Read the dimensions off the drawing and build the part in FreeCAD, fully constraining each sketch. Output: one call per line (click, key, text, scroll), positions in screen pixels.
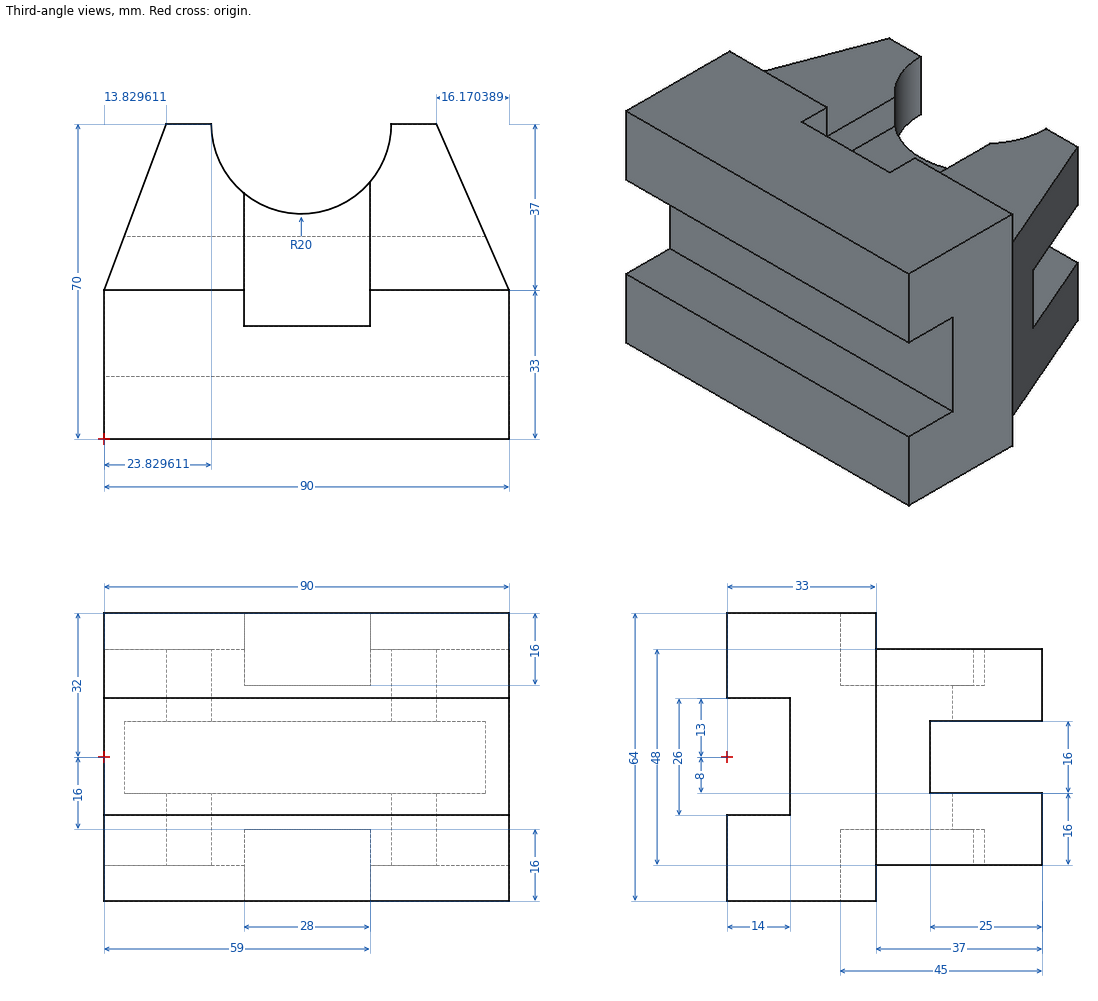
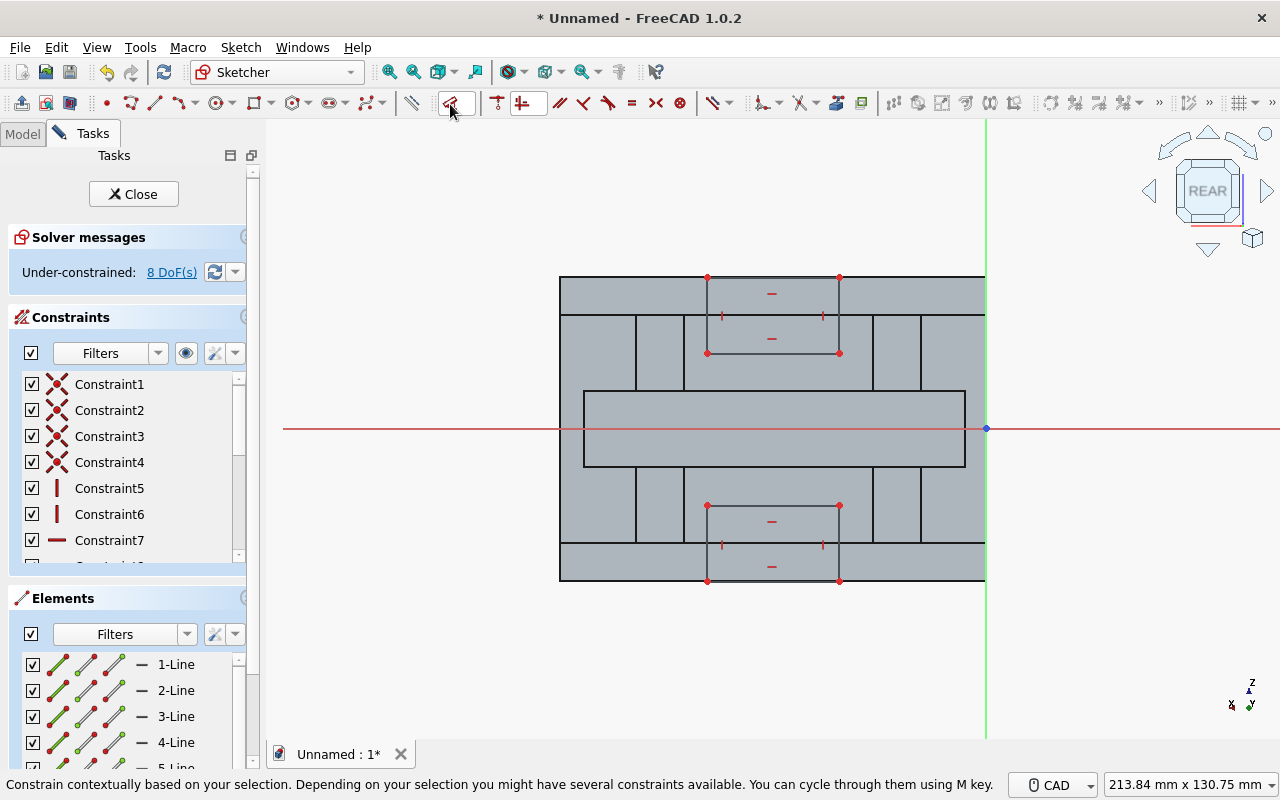
click(707, 529)
click(673, 544)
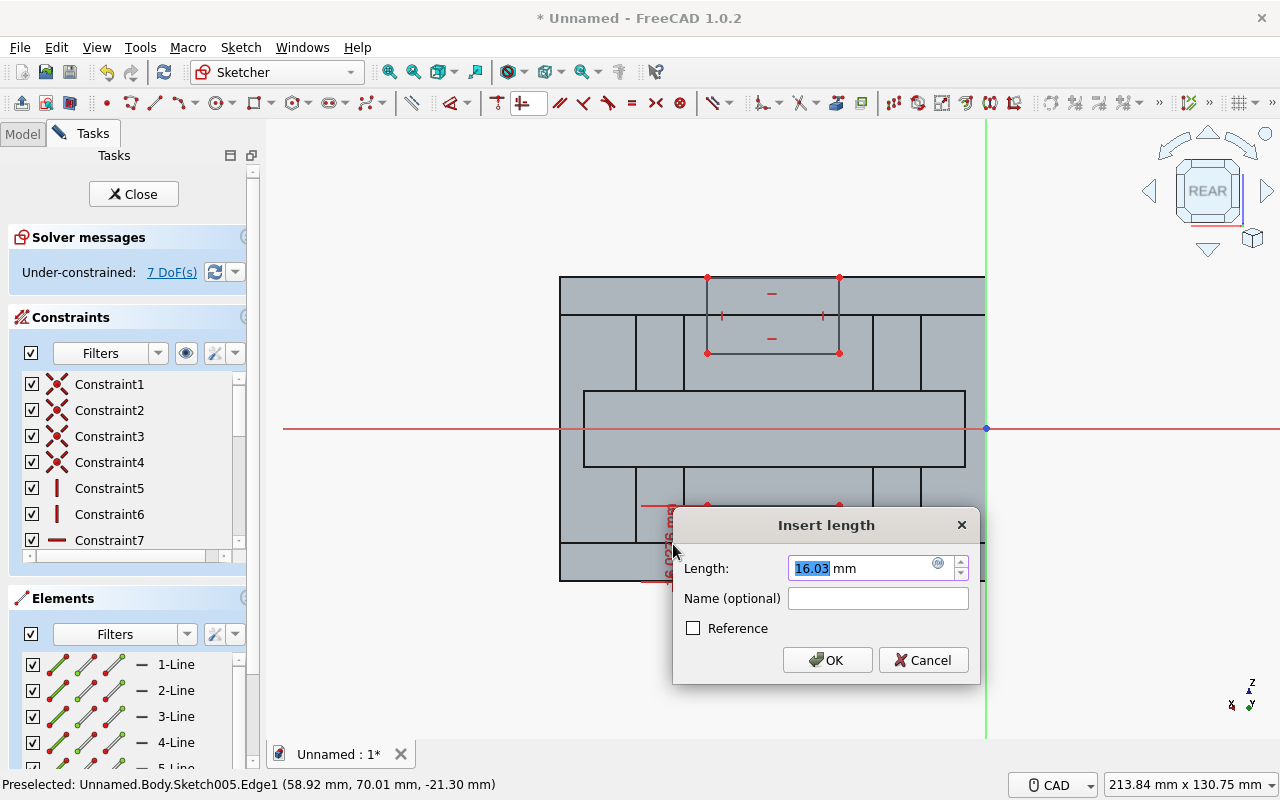
text(16)
key(Return)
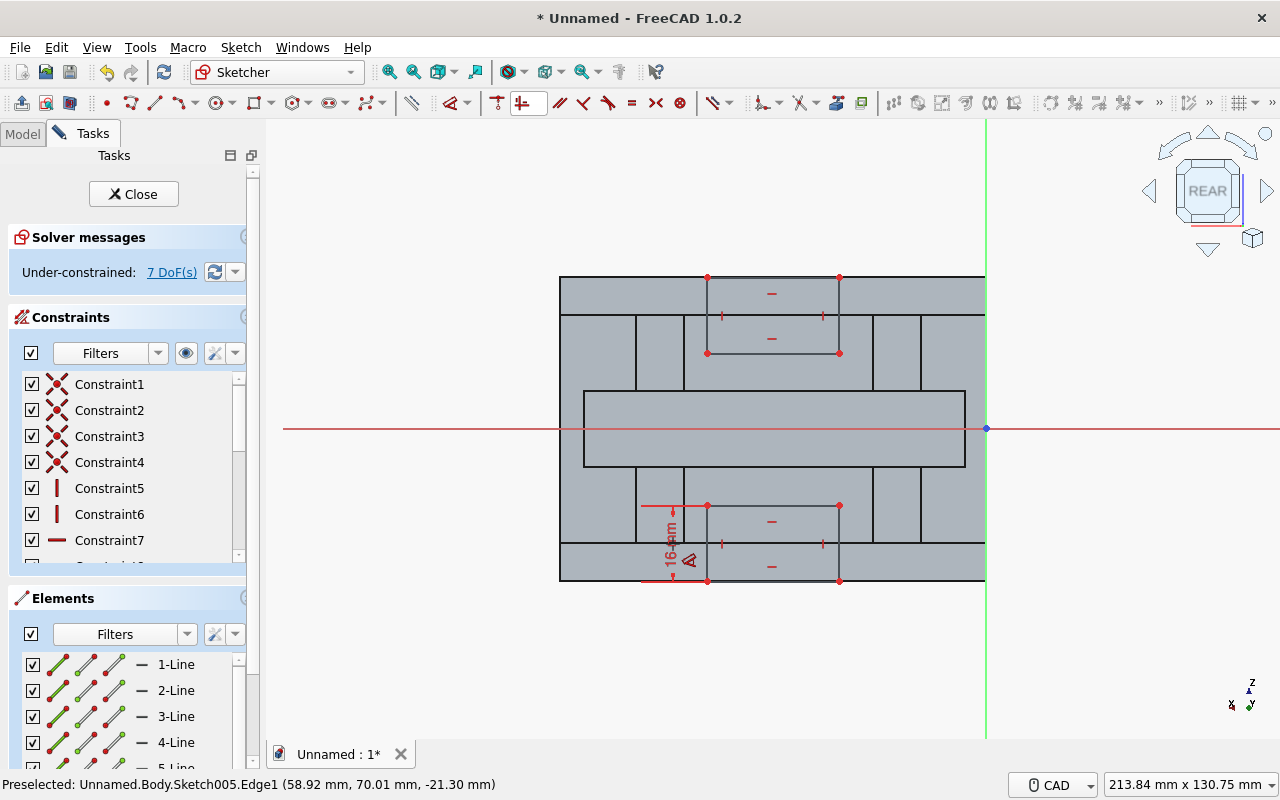
click(747, 582)
click(773, 616)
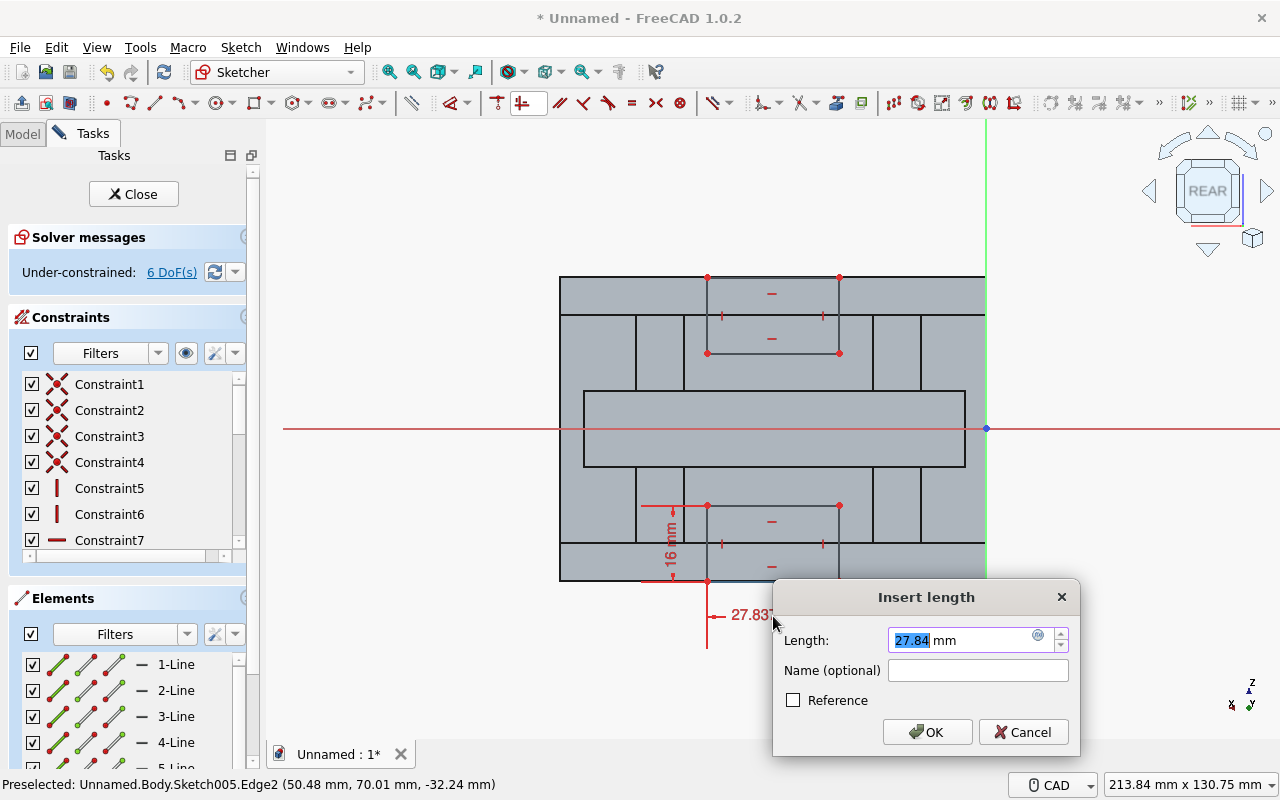
text(28)
key(Return)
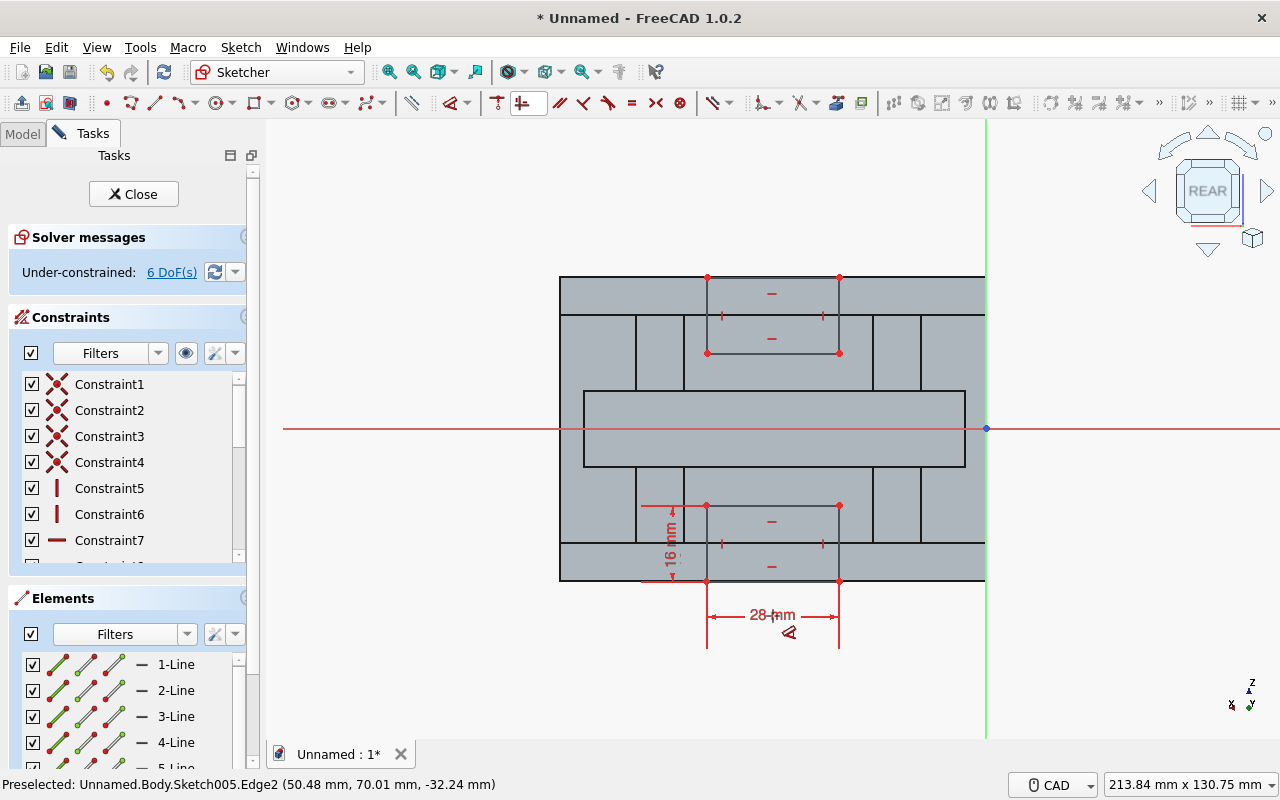
click(707, 301)
click(673, 316)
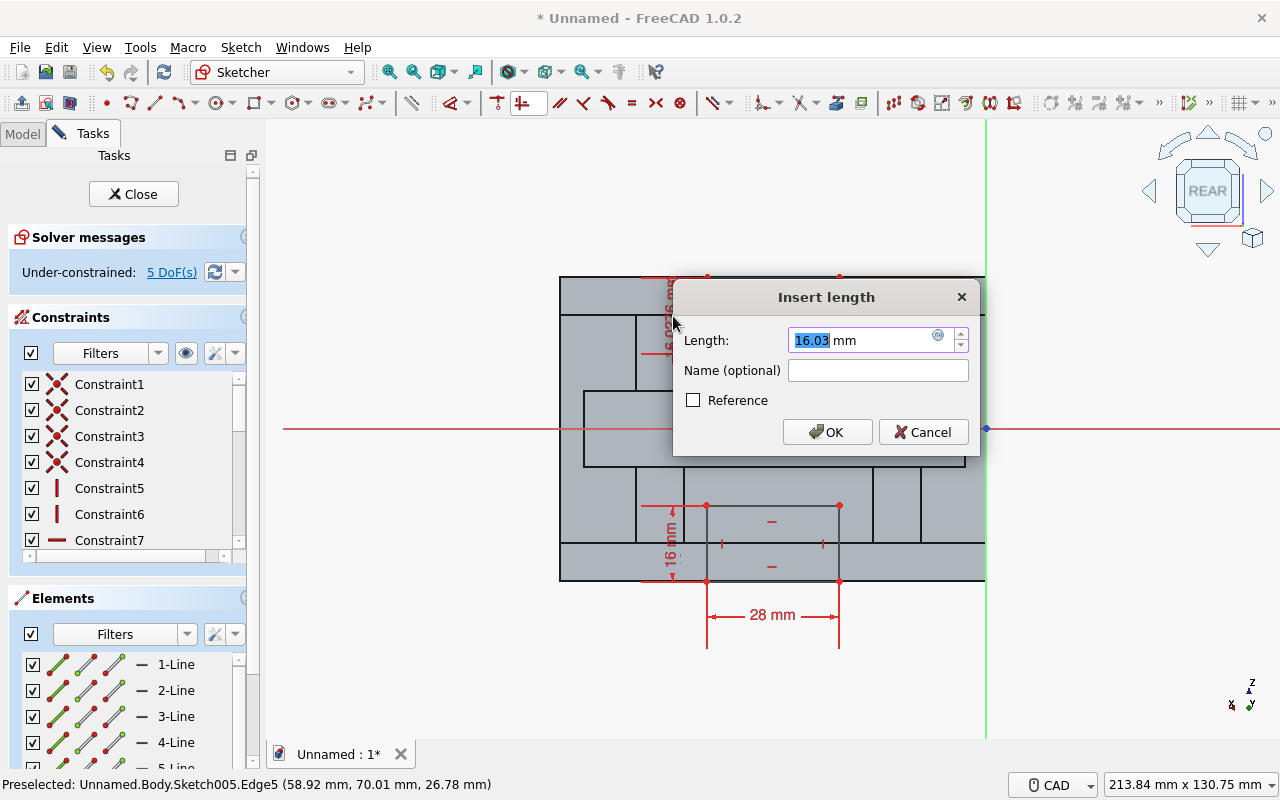
text(16)
key(Return)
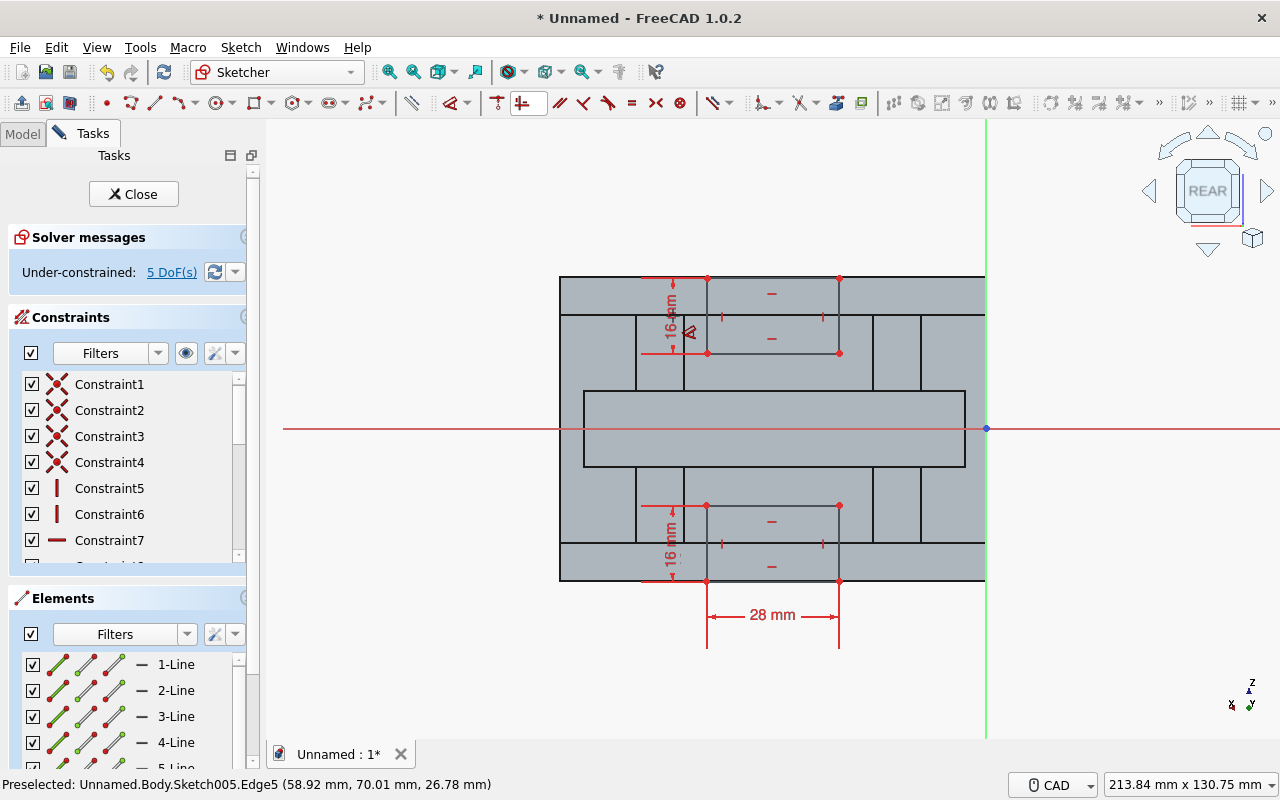
click(747, 354)
click(773, 320)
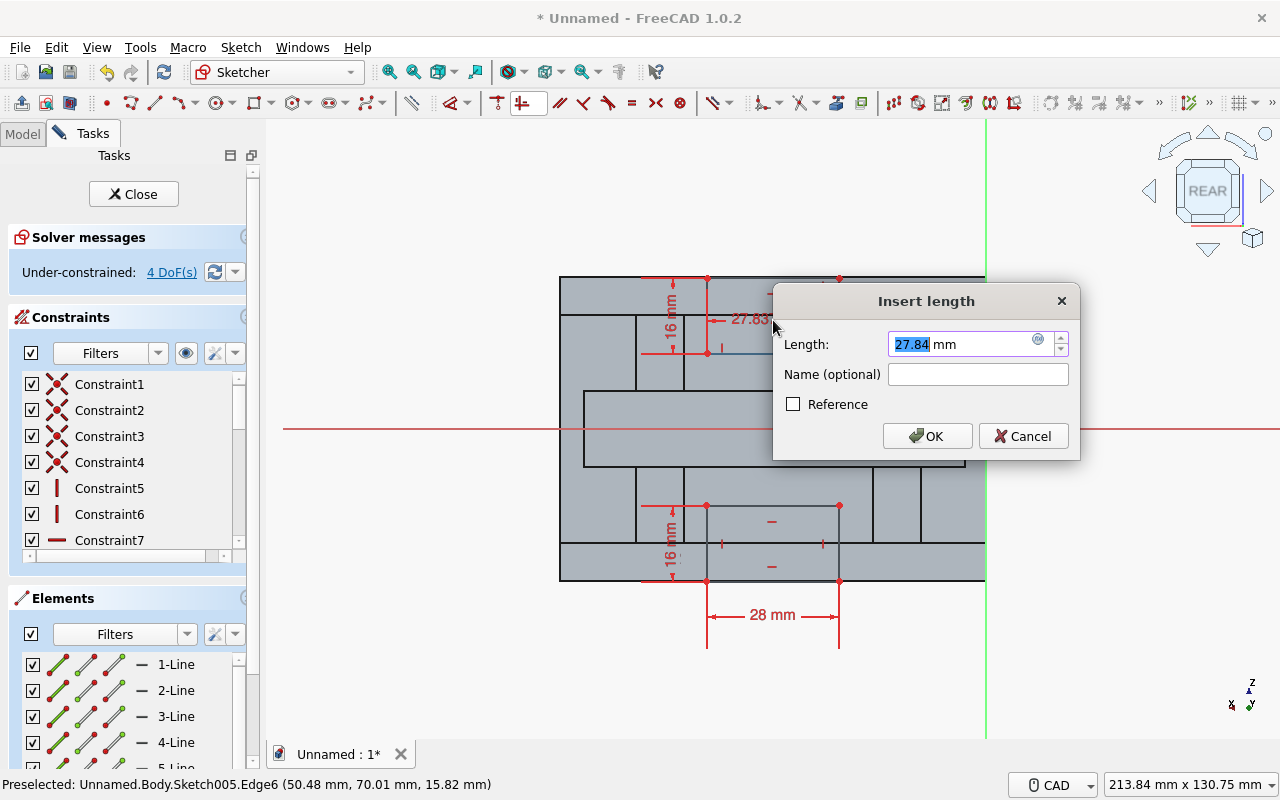
text(28)
key(Return)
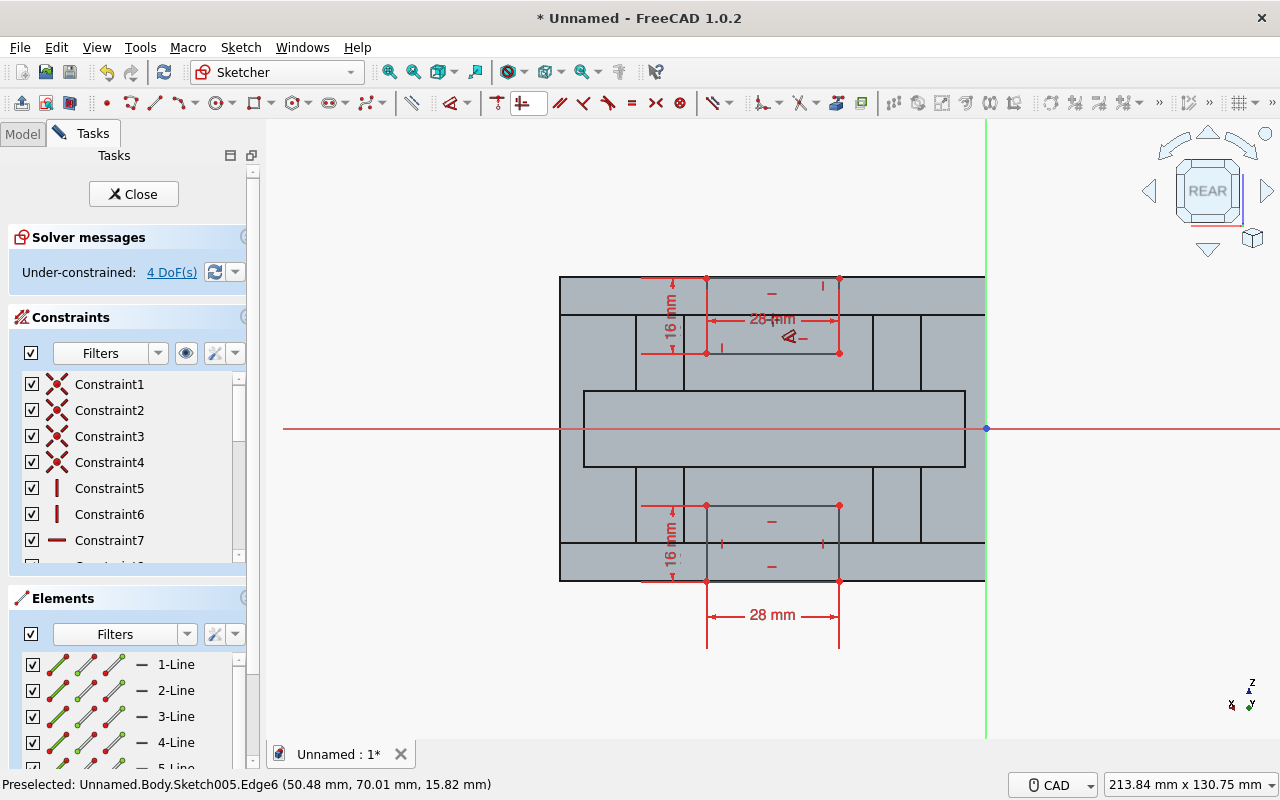
click(707, 506)
click(782, 540)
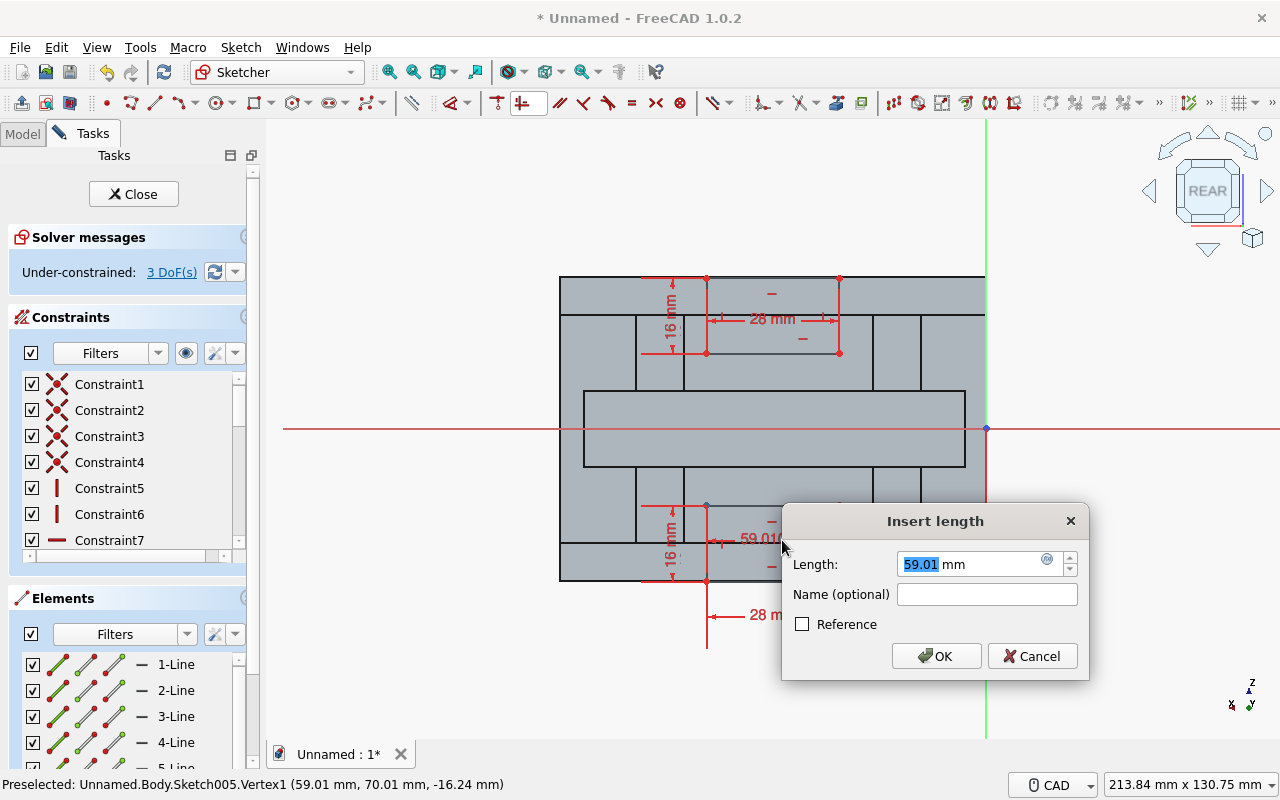
text(59)
key(Return)